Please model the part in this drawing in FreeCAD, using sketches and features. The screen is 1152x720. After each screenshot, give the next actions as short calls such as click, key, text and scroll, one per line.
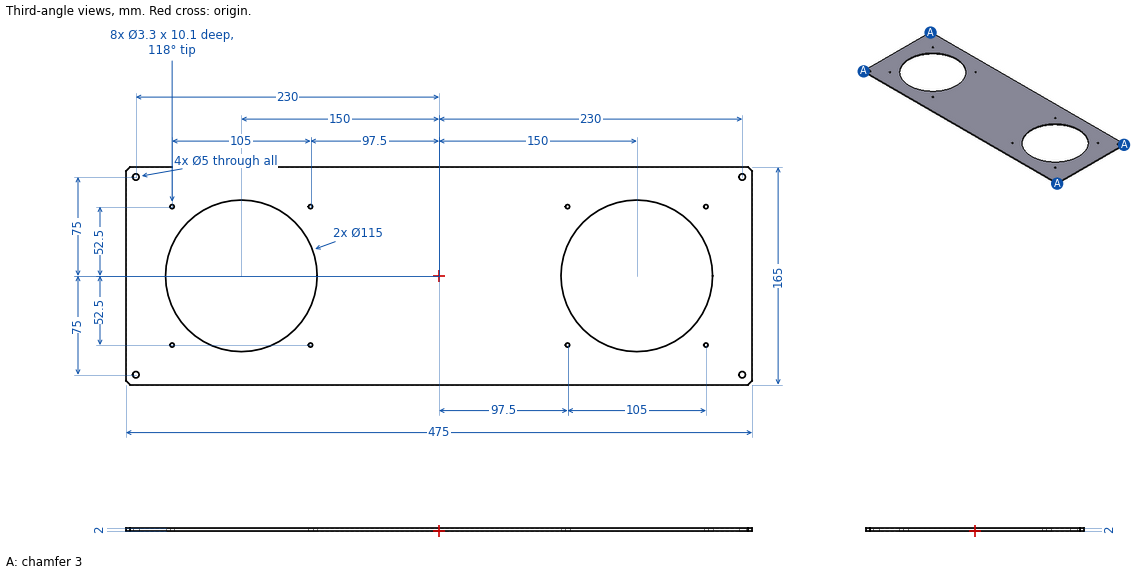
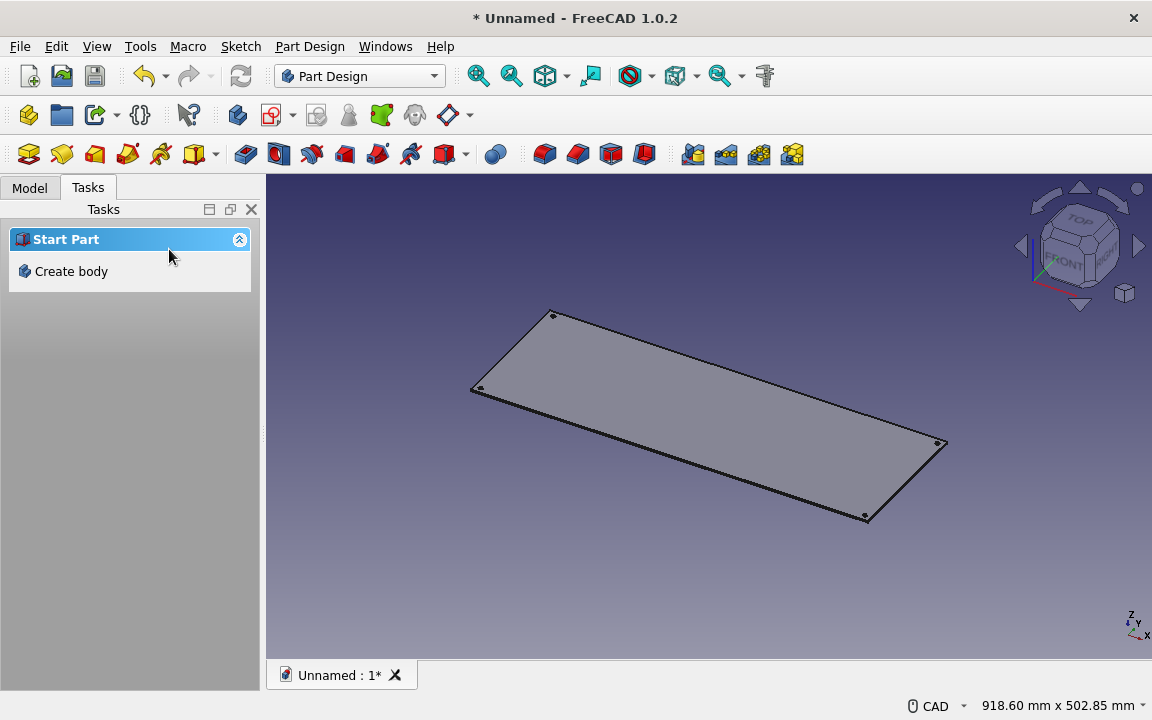
scroll(868, 521, up, 15)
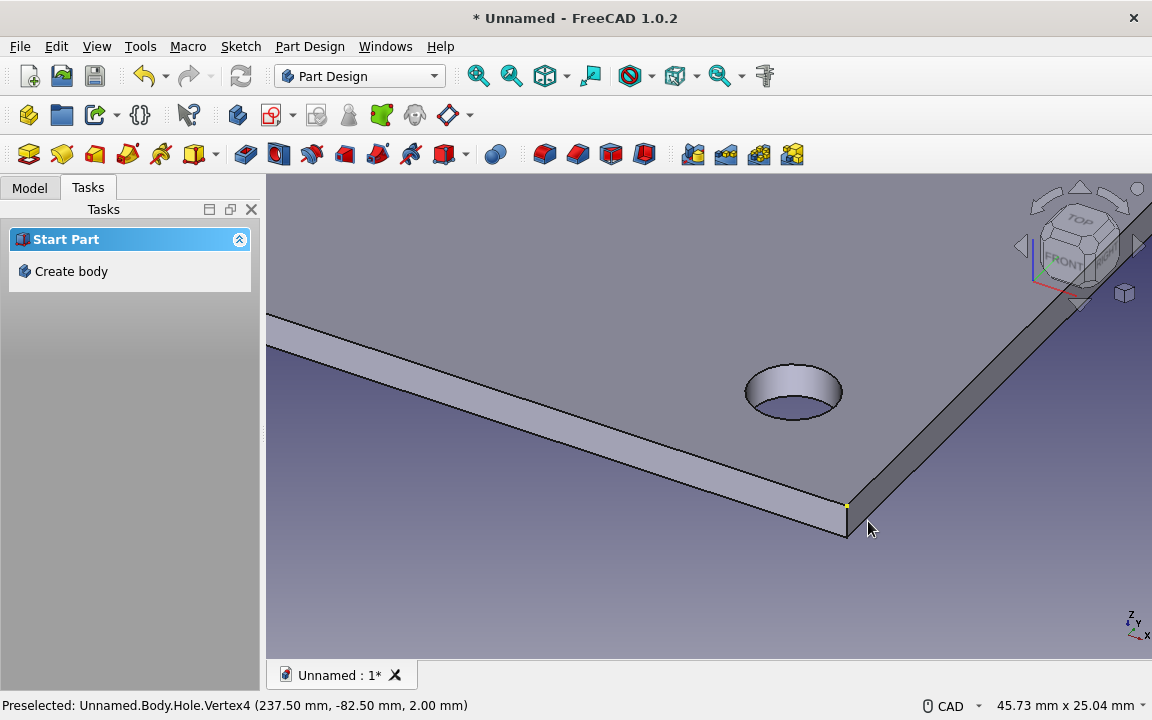
click(847, 521)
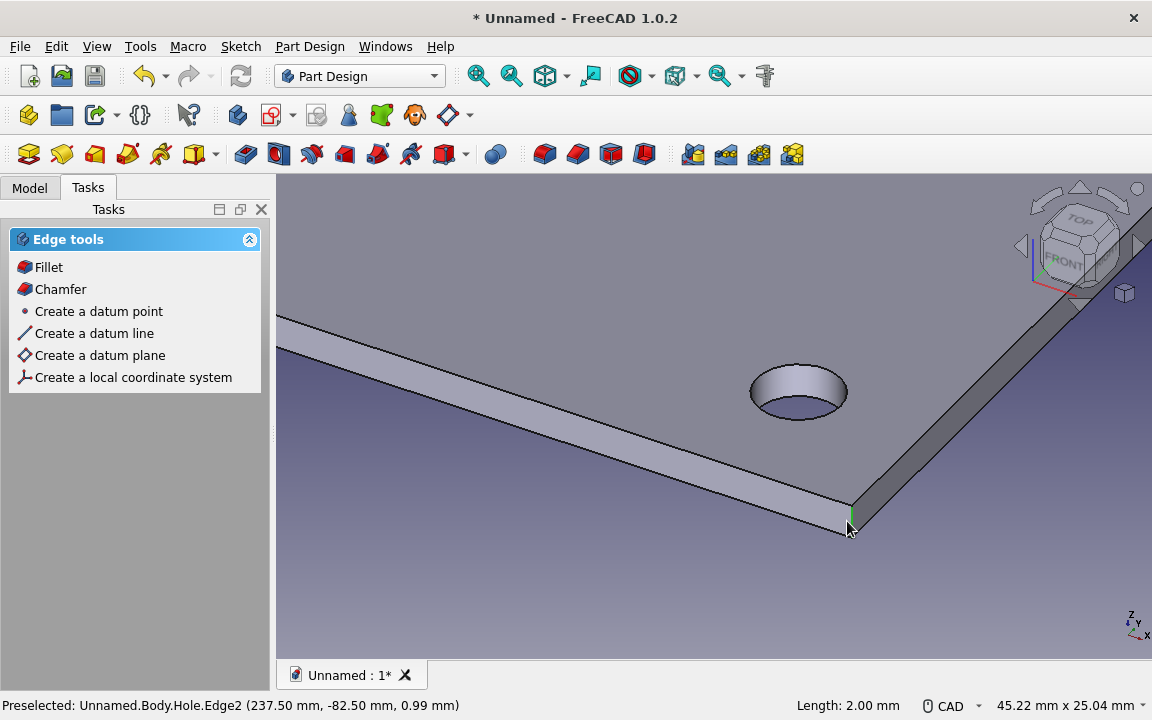
key(v)
key(f)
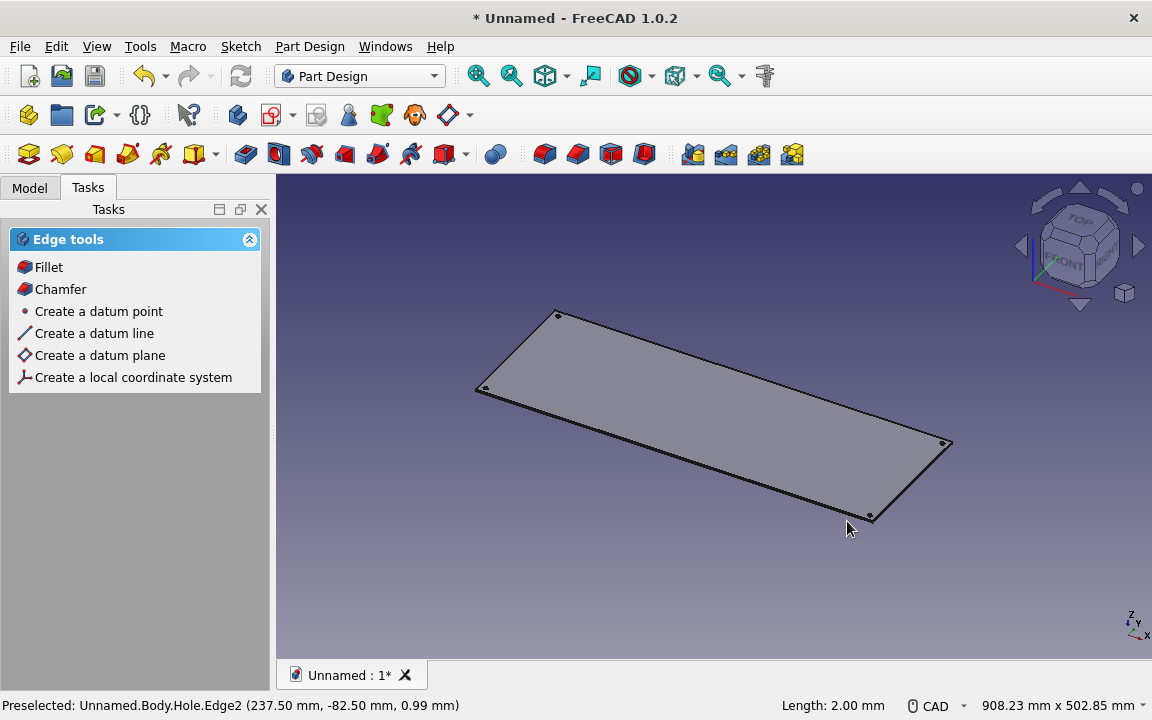
key(0)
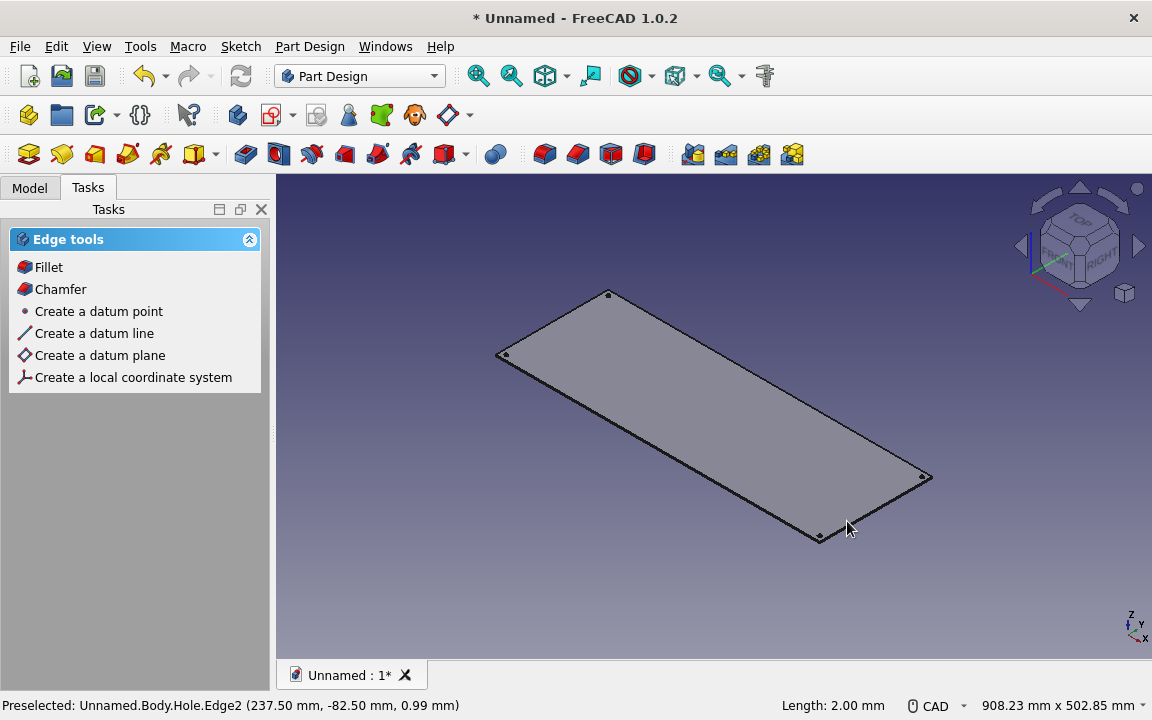
scroll(496, 354, up, 15)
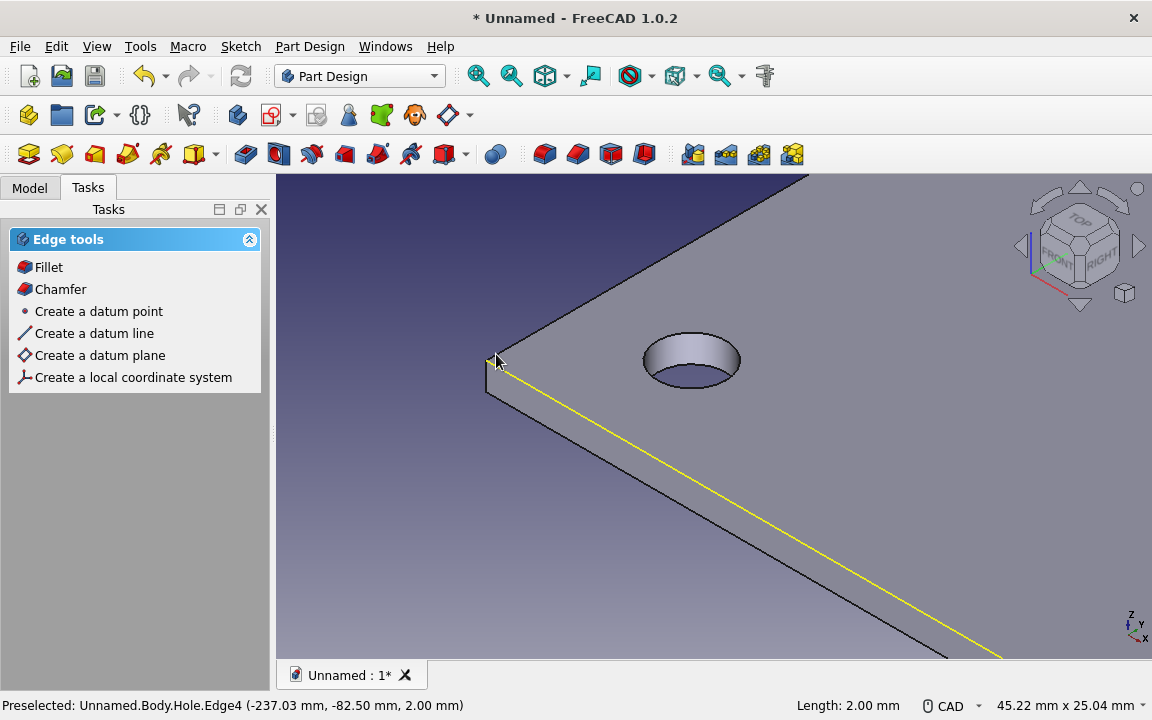
click(479, 76)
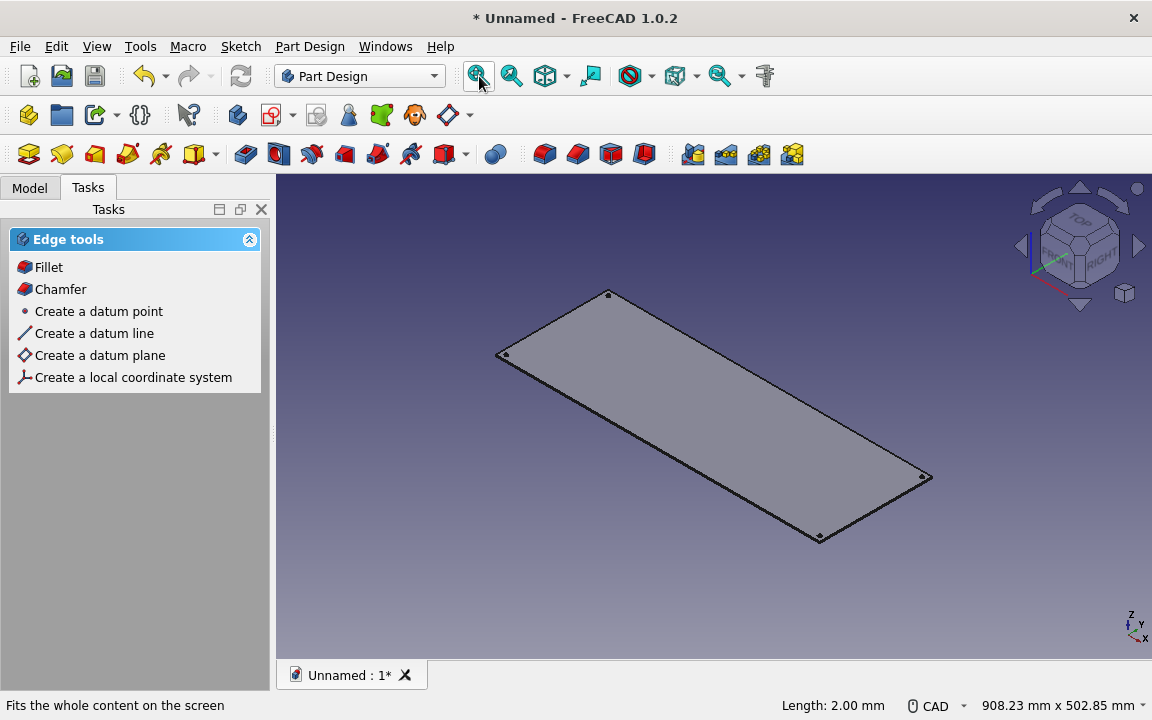
key(2)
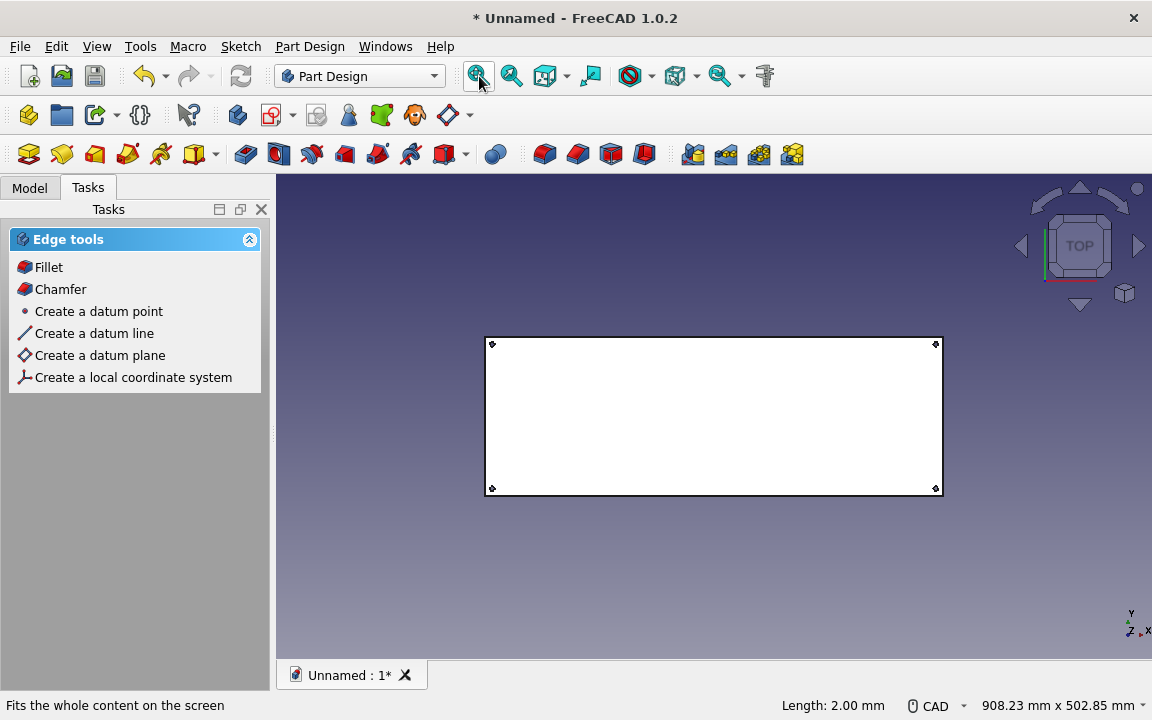
scroll(485, 495, up, 15)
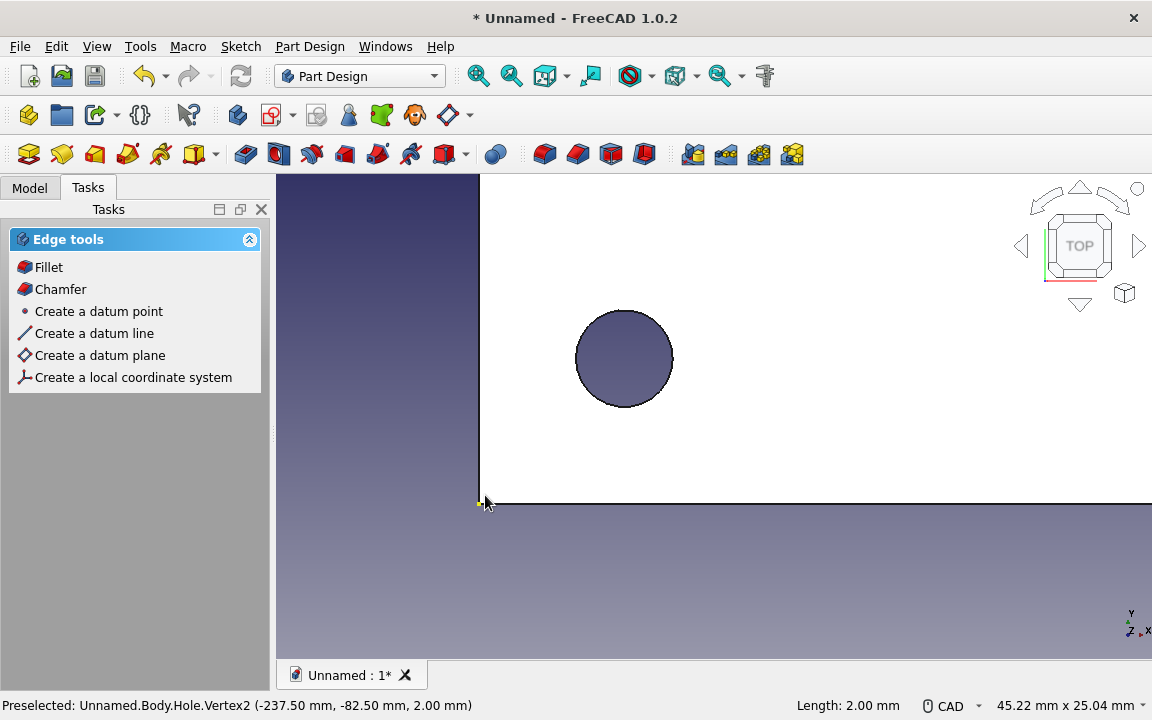
key(v)
key(f)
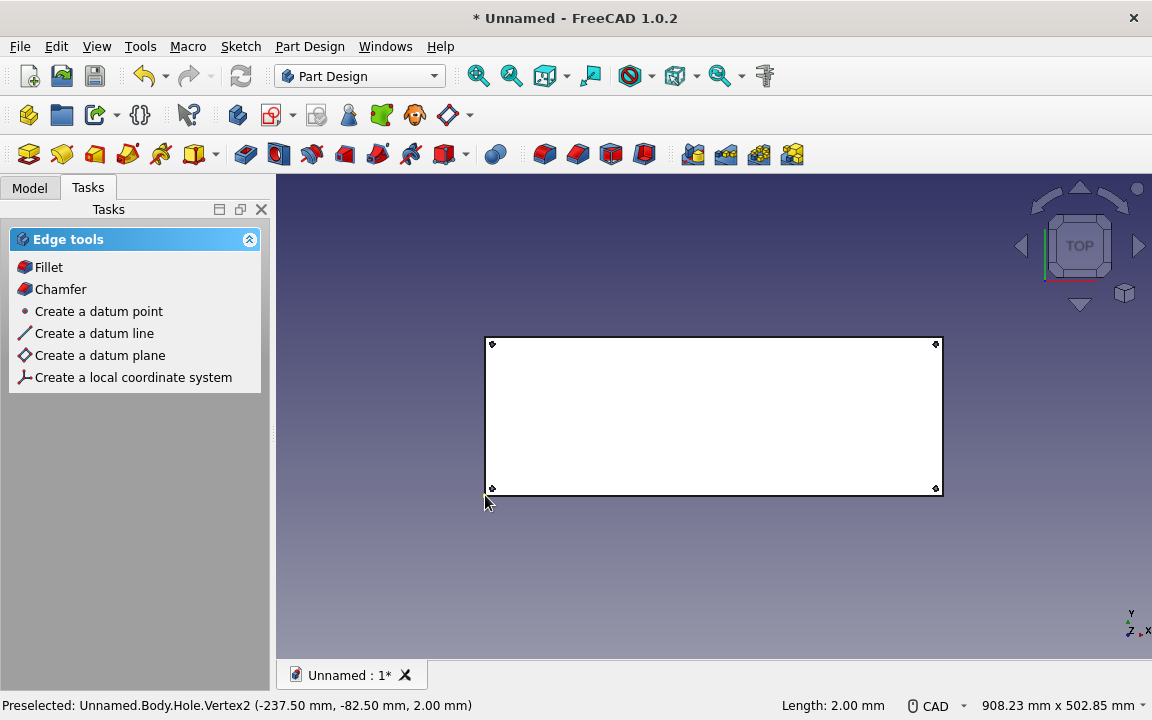
key(1)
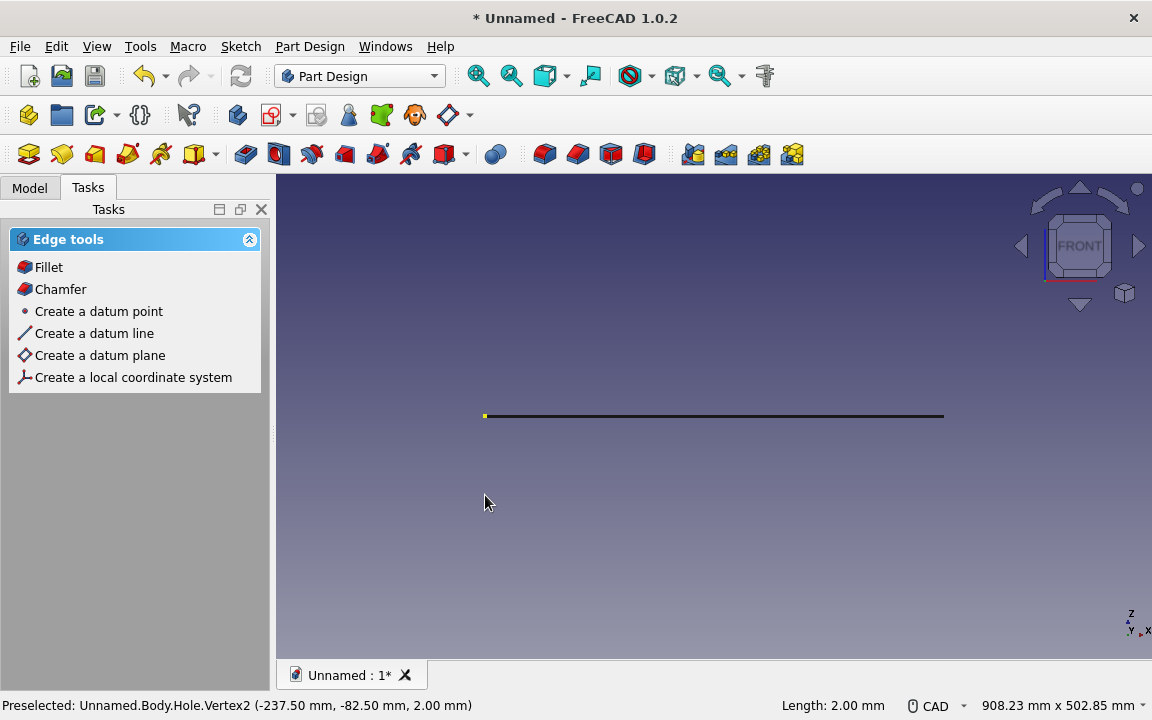
scroll(485, 415, up, 15)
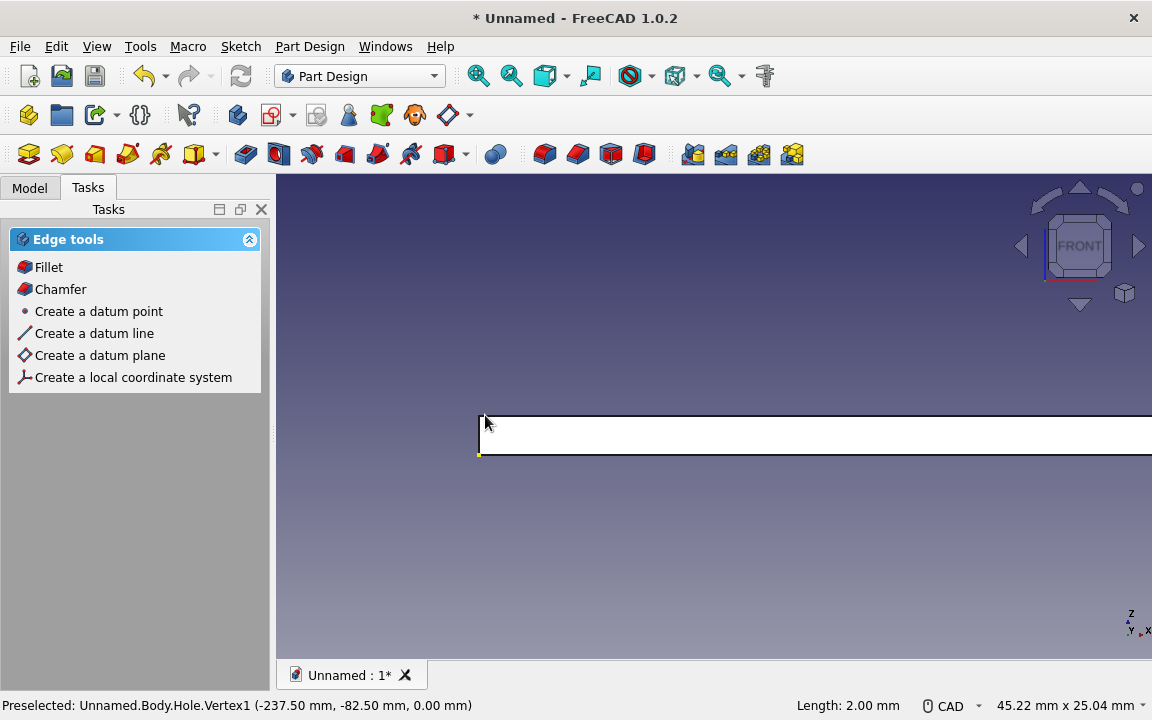
click(479, 435, ctrl)